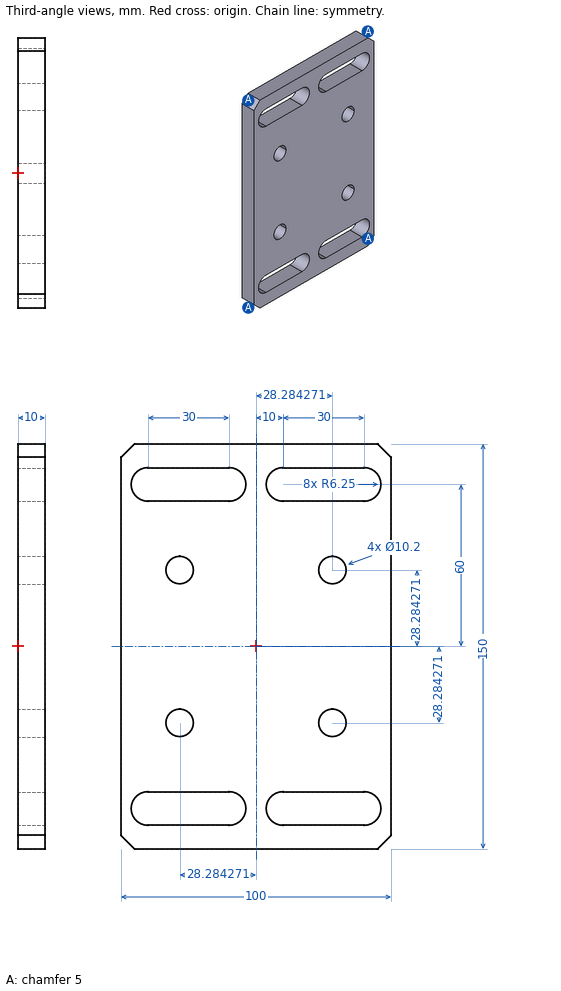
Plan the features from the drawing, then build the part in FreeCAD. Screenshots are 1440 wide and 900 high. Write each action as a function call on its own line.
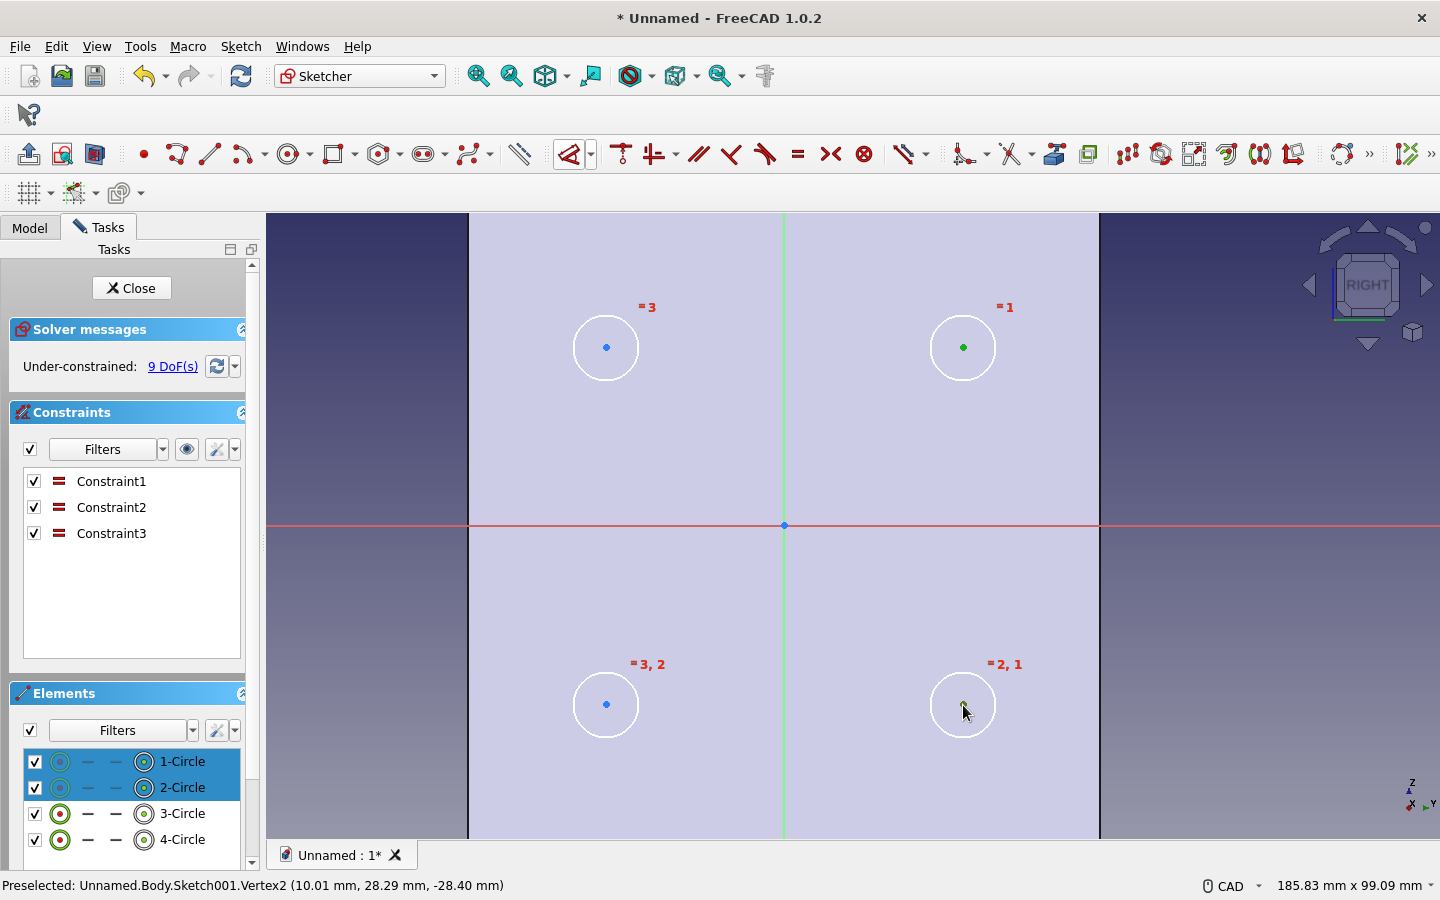
key(v)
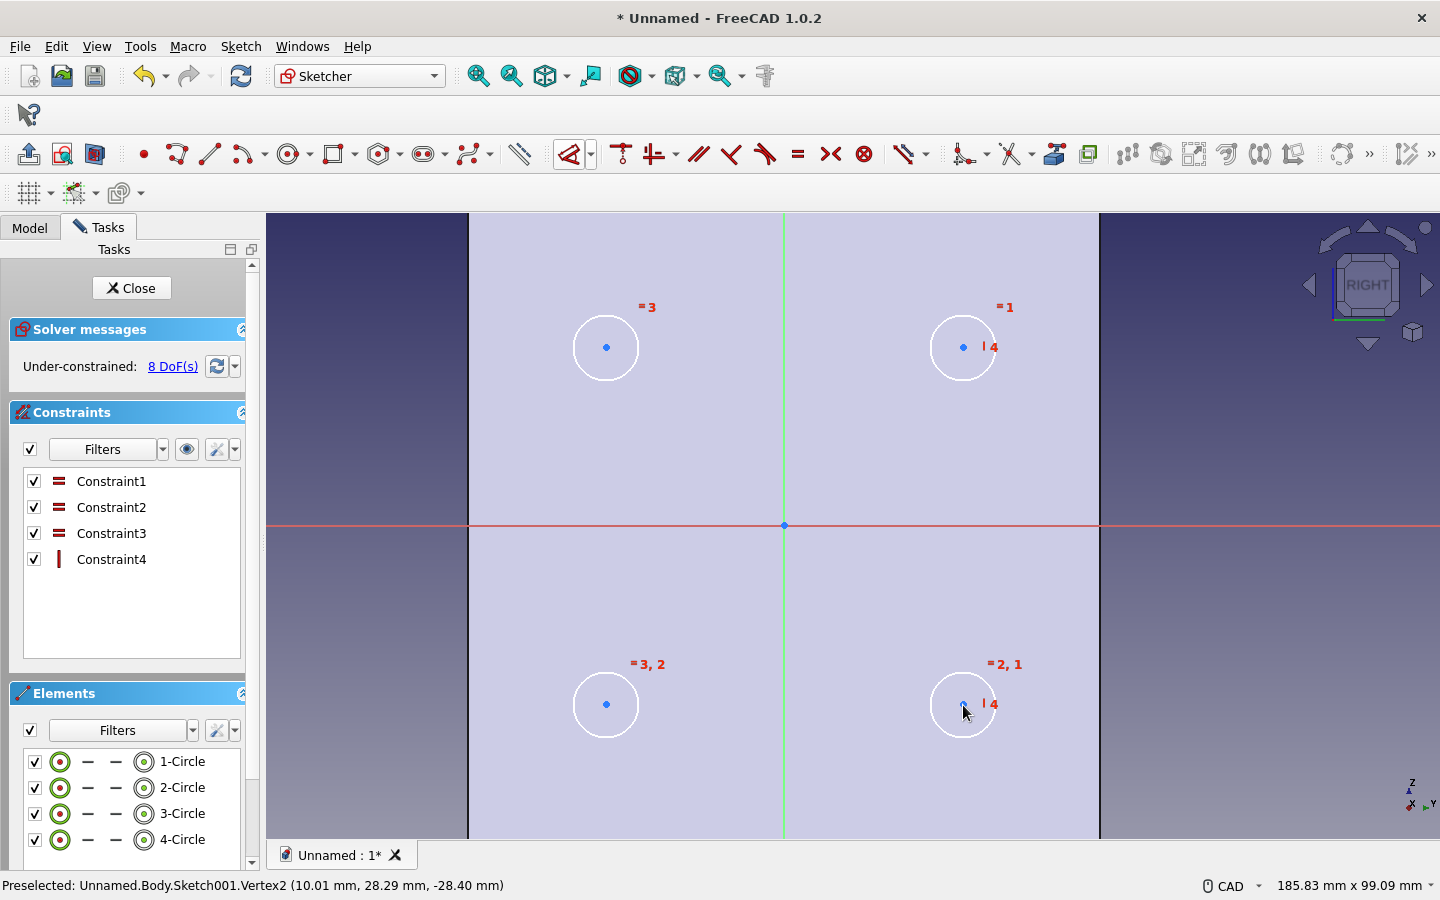
click(963, 705)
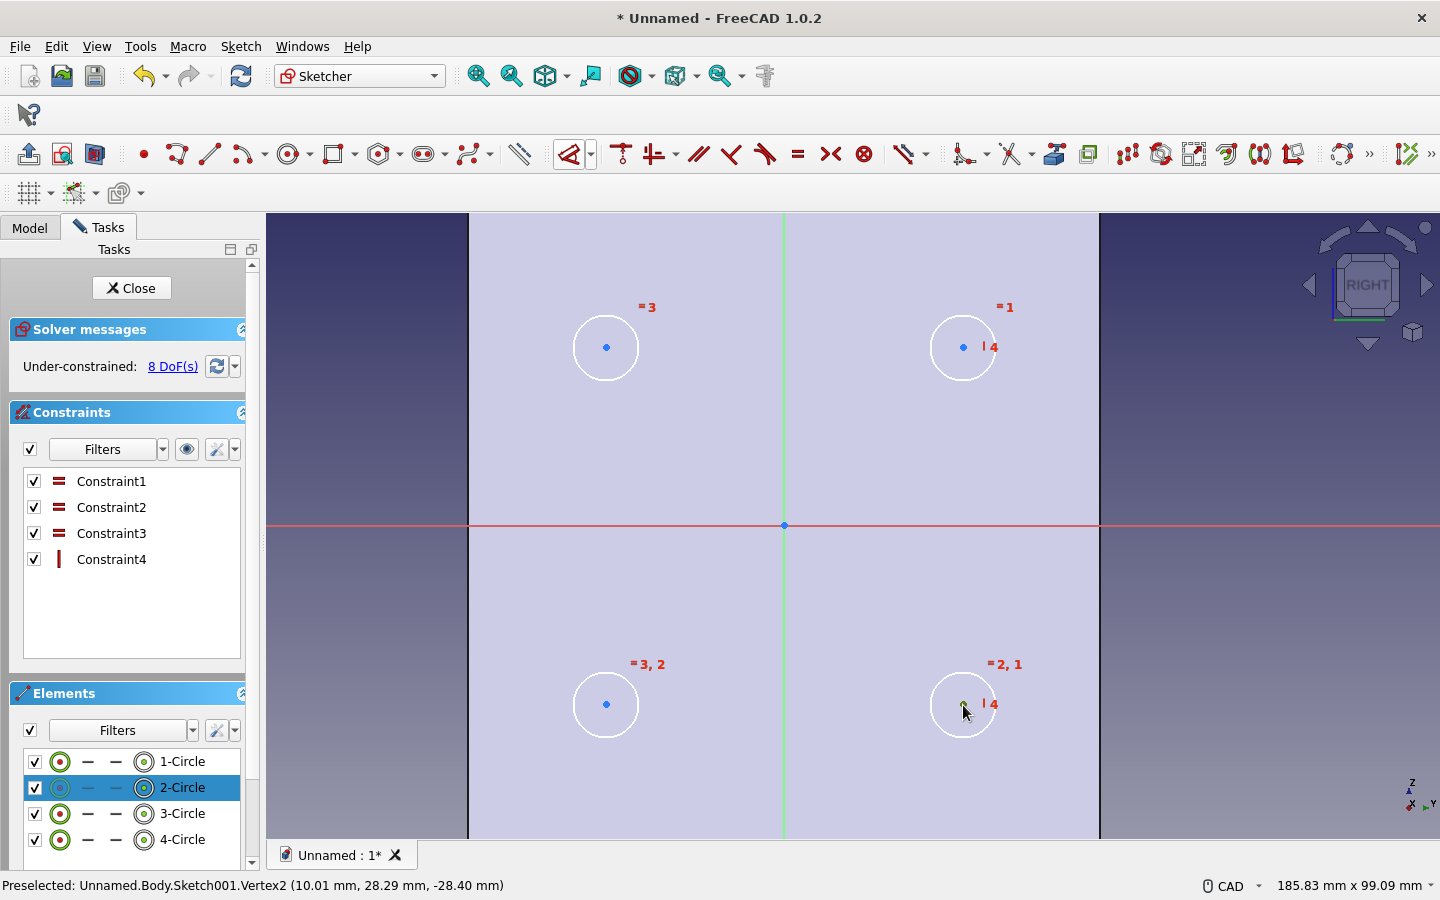
click(606, 705)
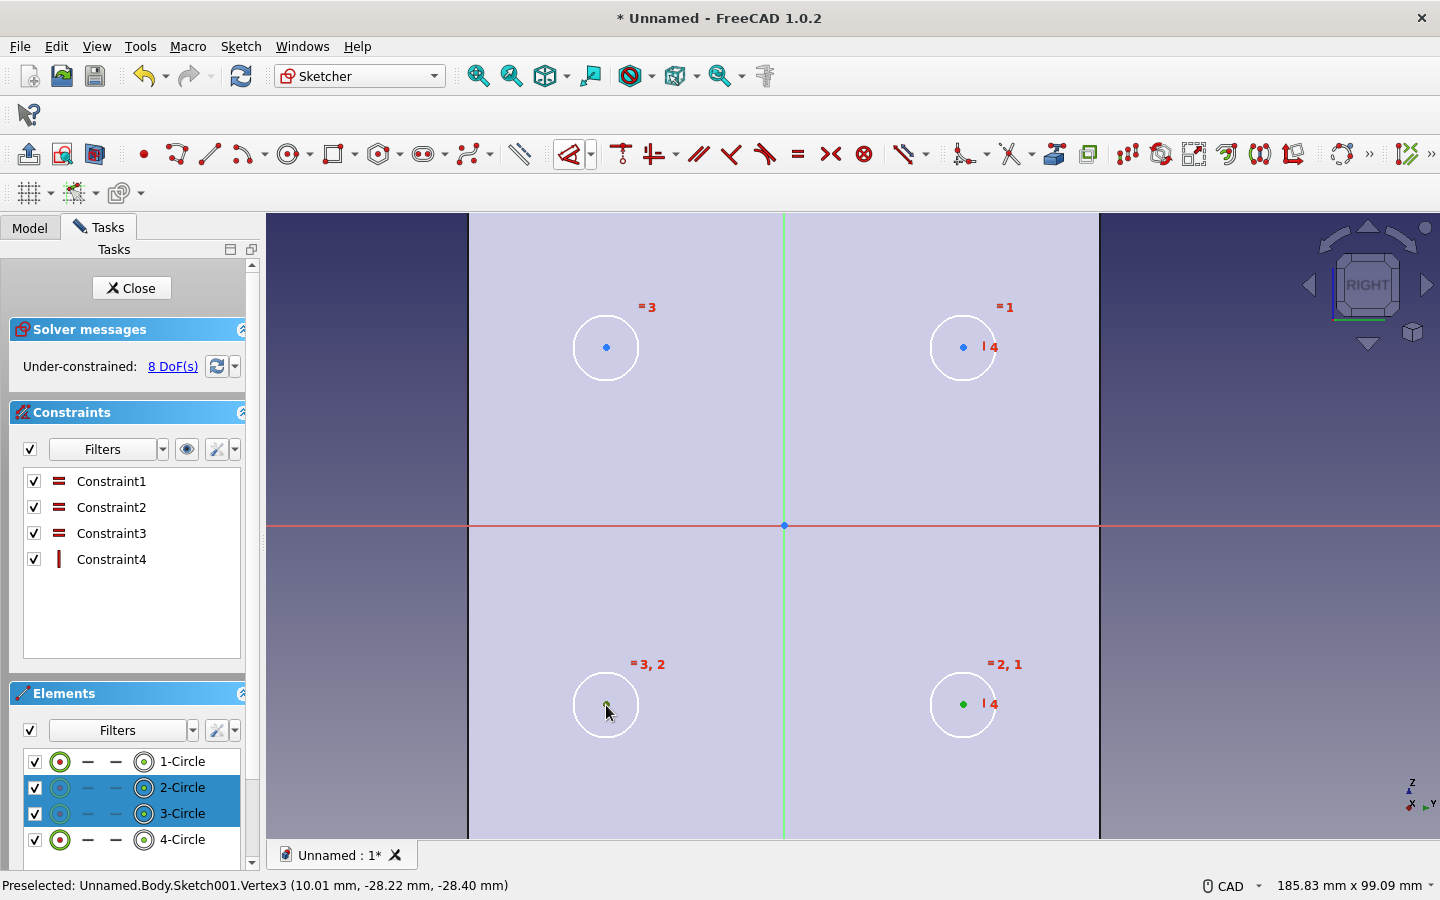
click(676, 154)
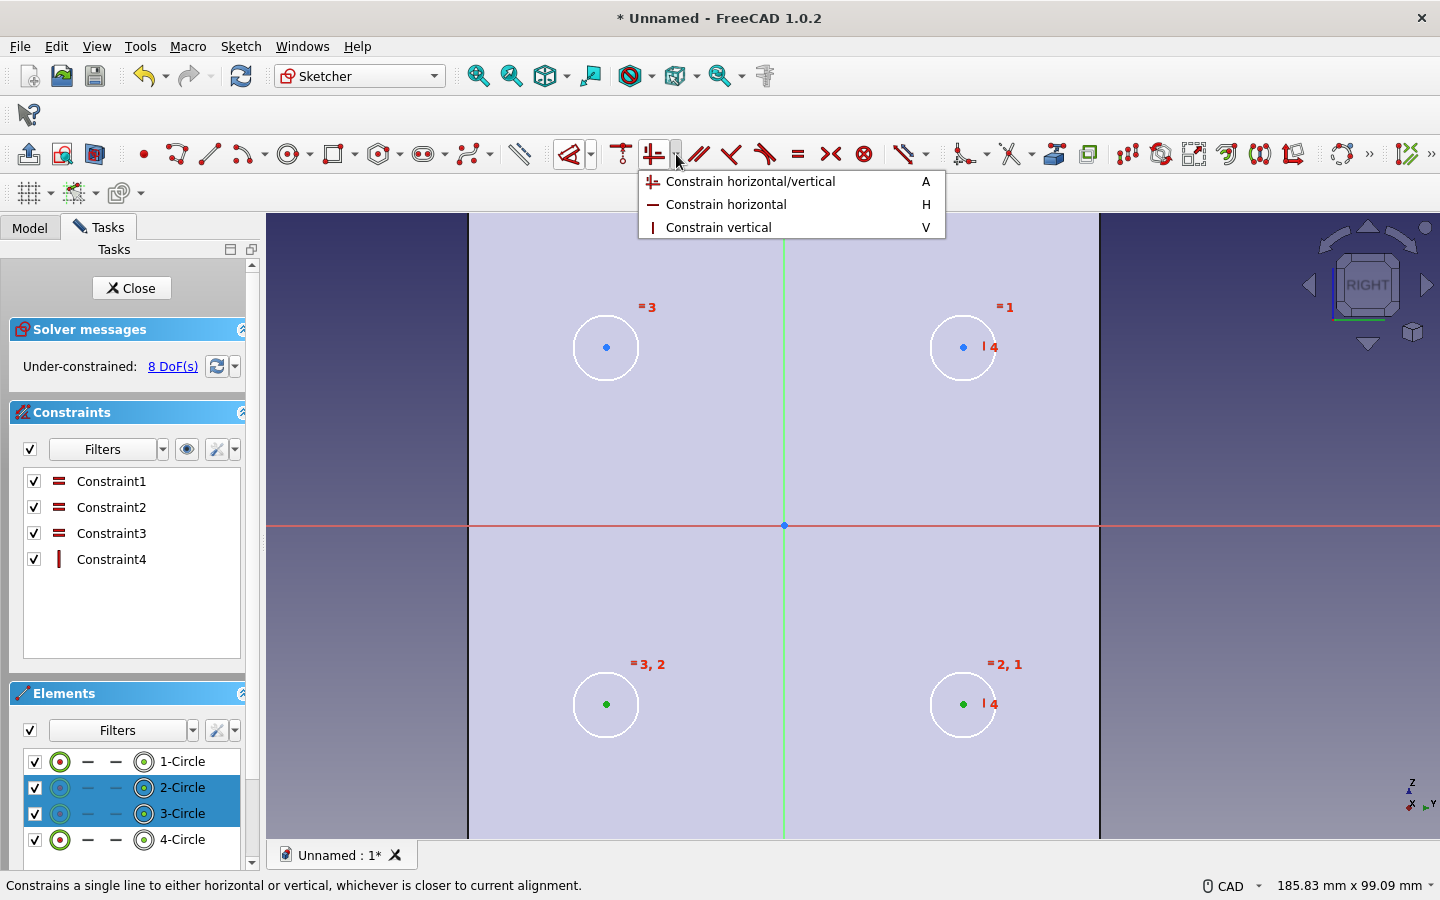
click(792, 204)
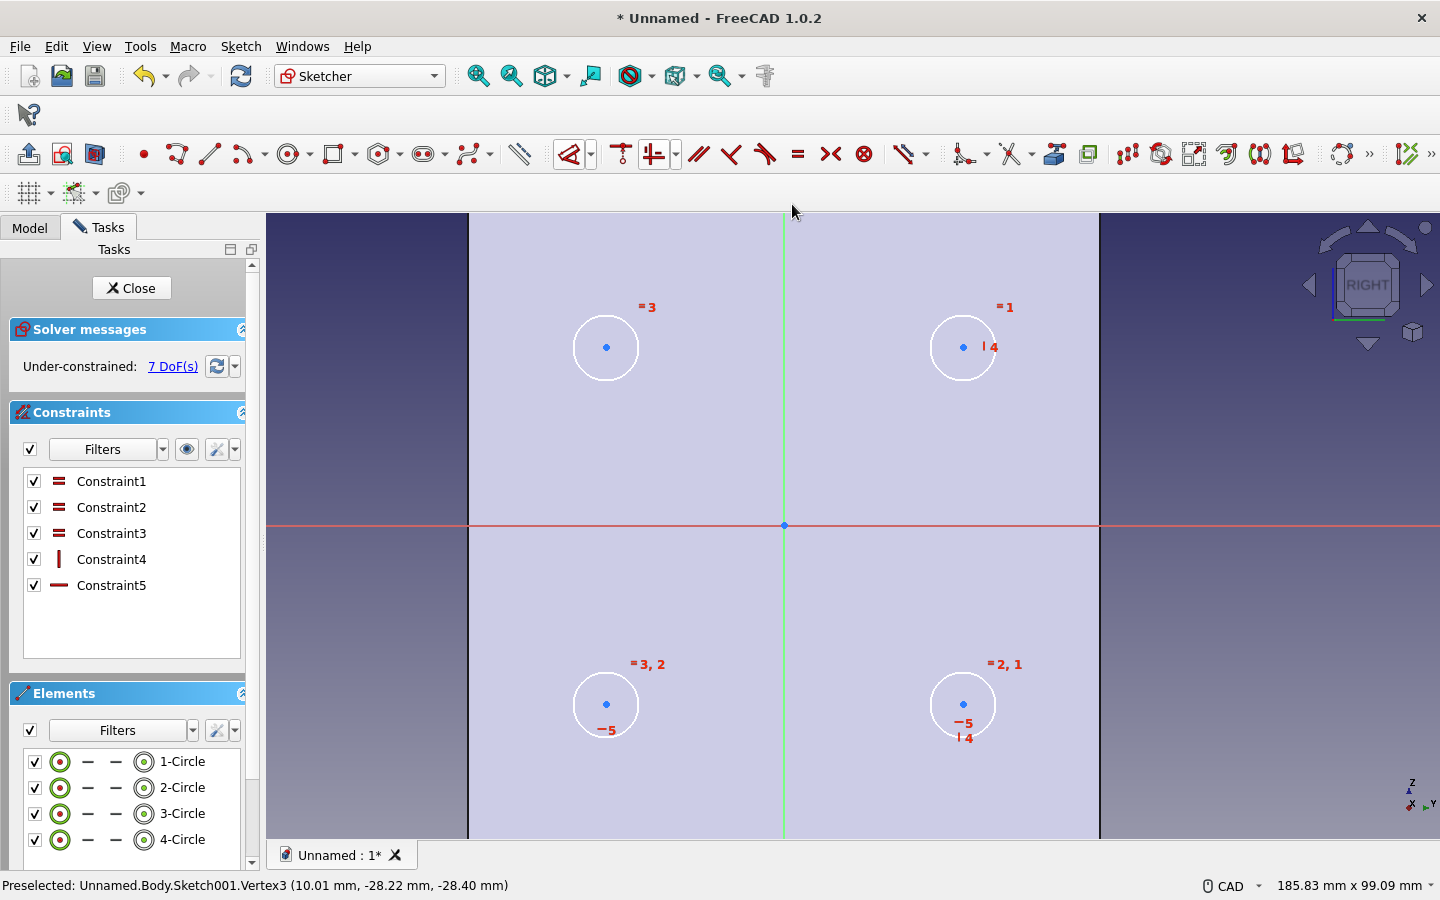
click(606, 705)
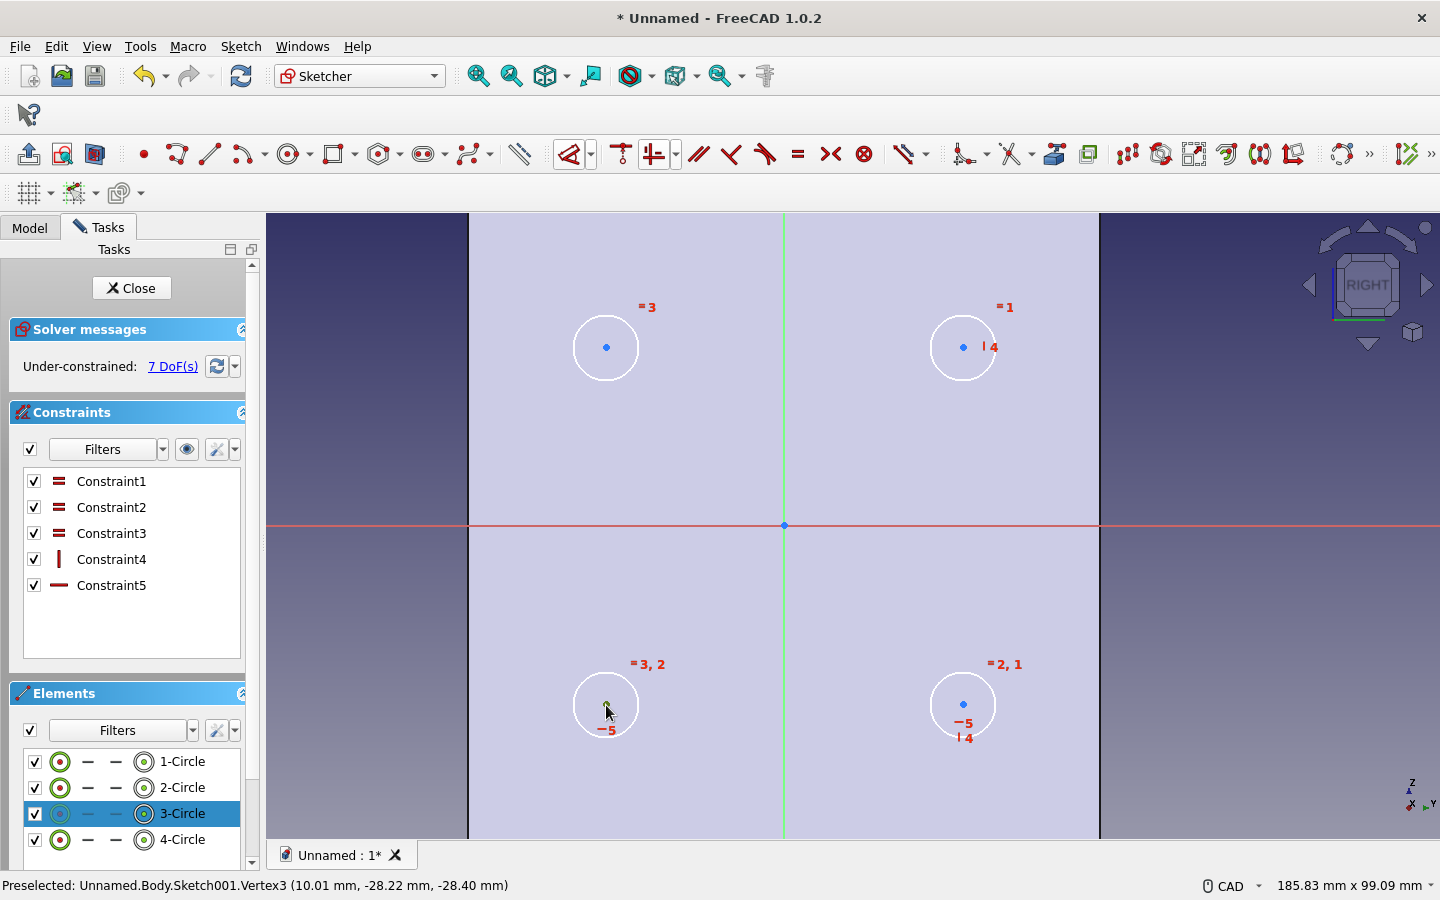
click(606, 348)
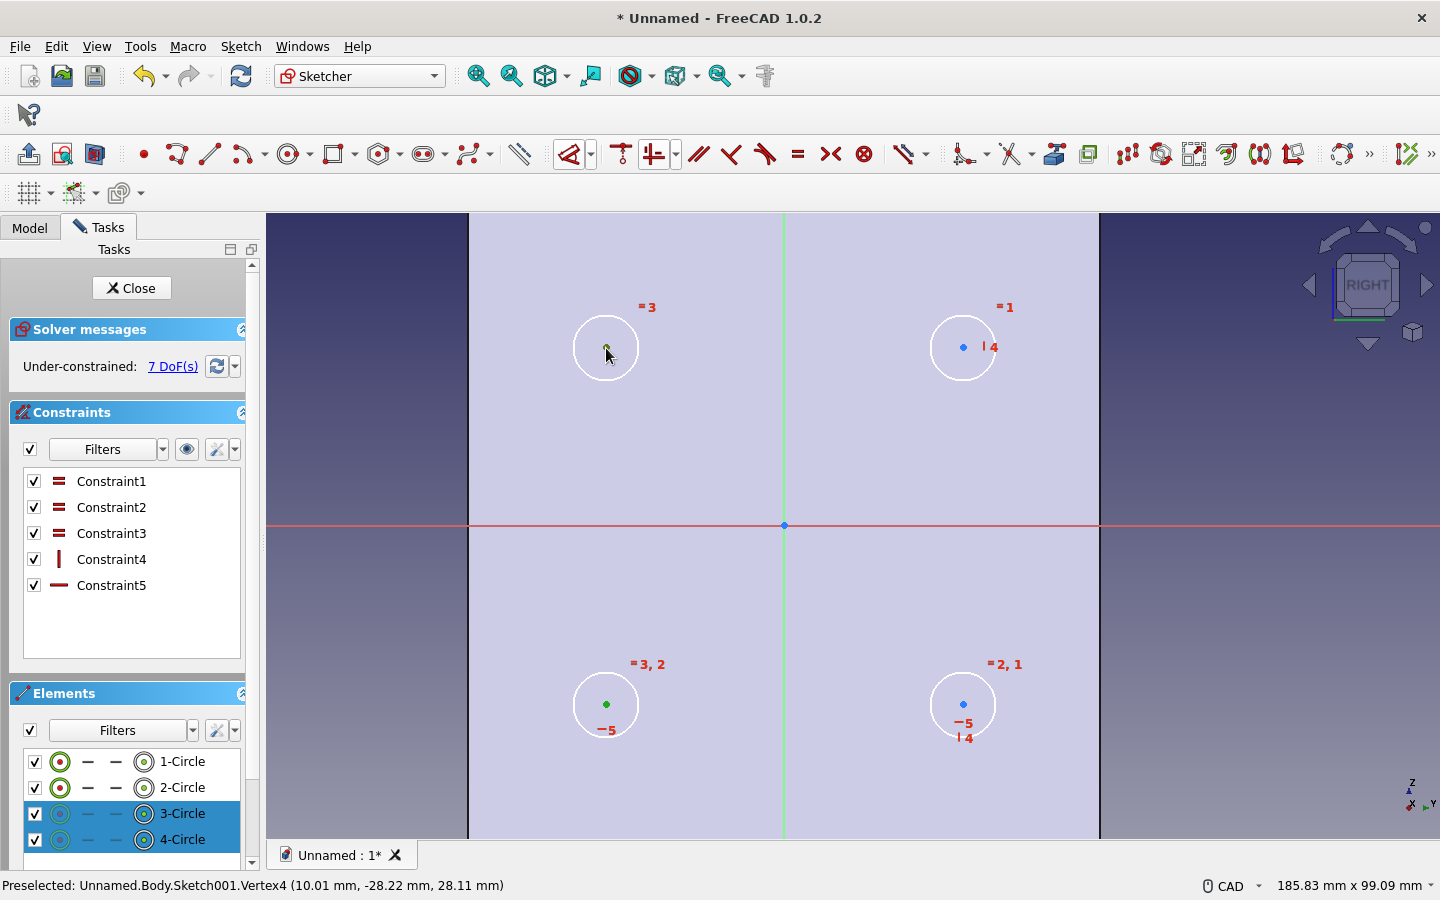
key(v)